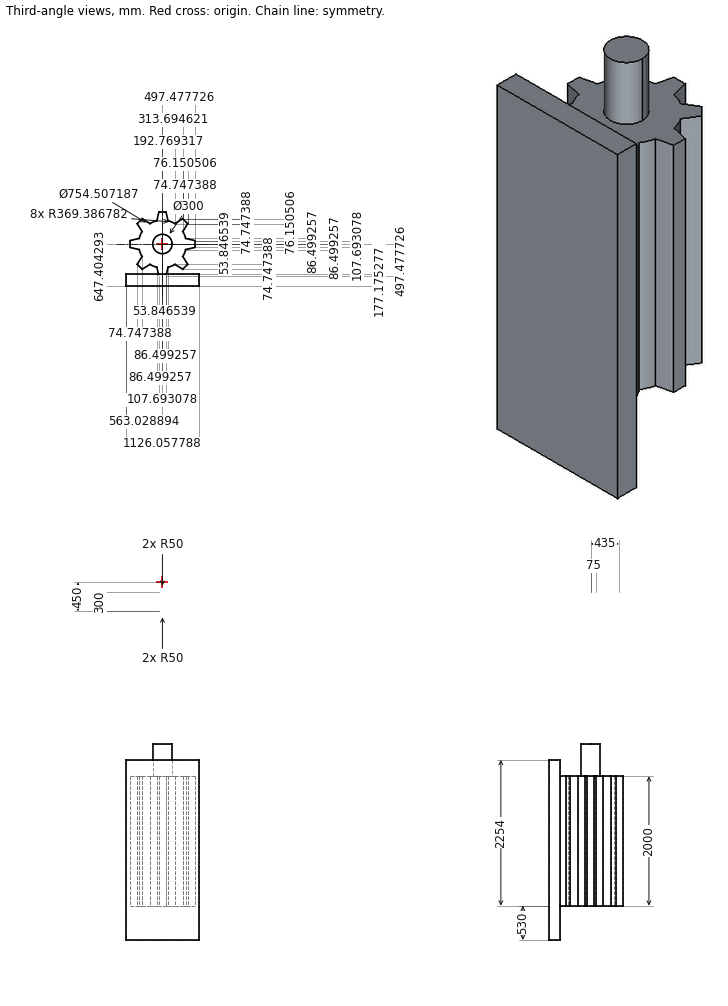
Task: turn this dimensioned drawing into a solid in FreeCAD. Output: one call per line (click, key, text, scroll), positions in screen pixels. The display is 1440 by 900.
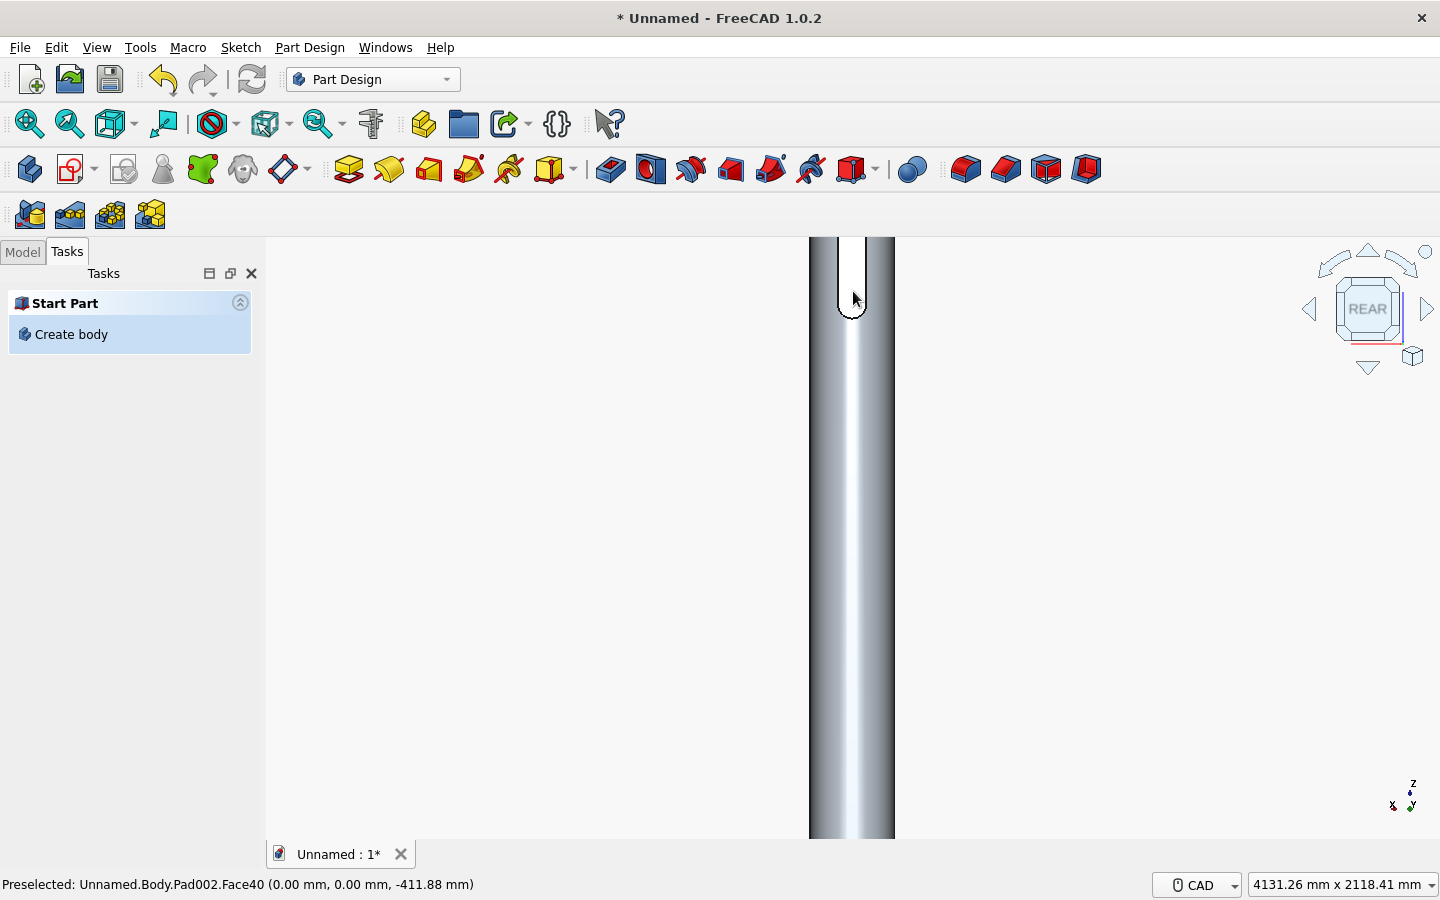
click(852, 293)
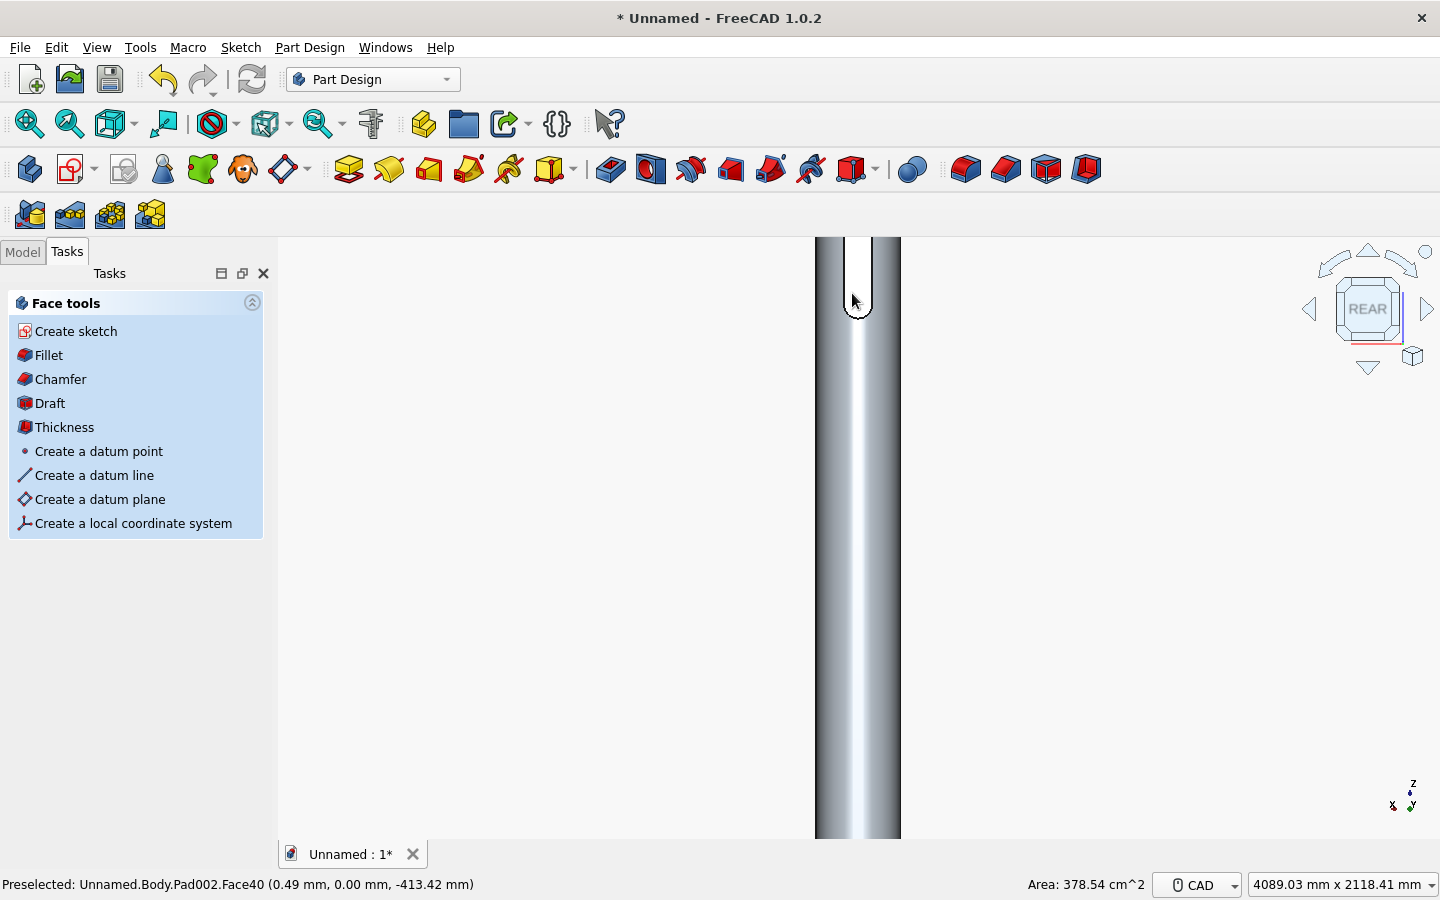
click(70, 170)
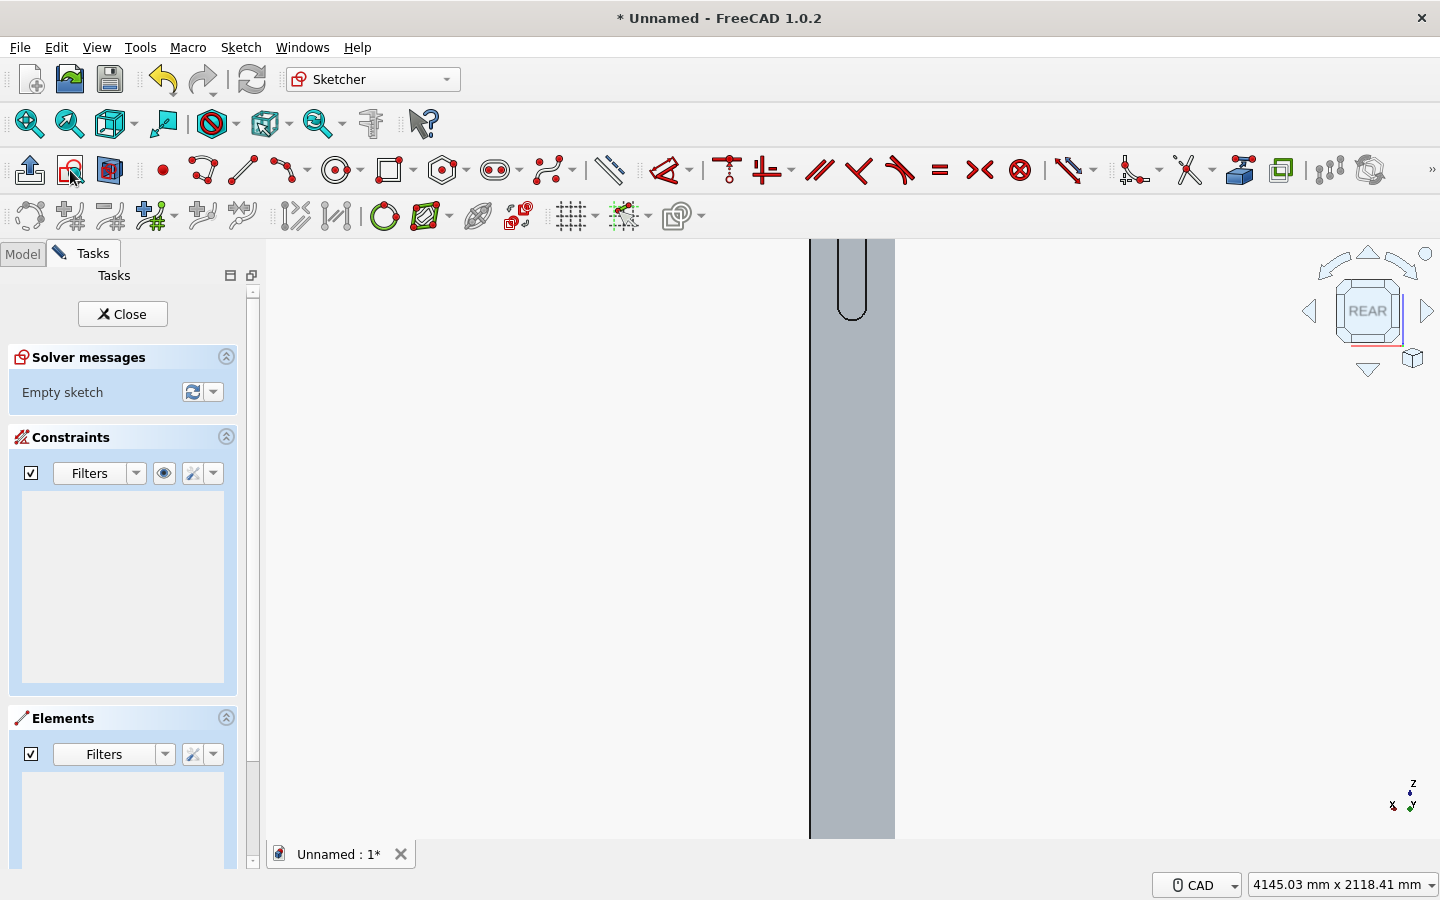
scroll(784, 539, down, 5)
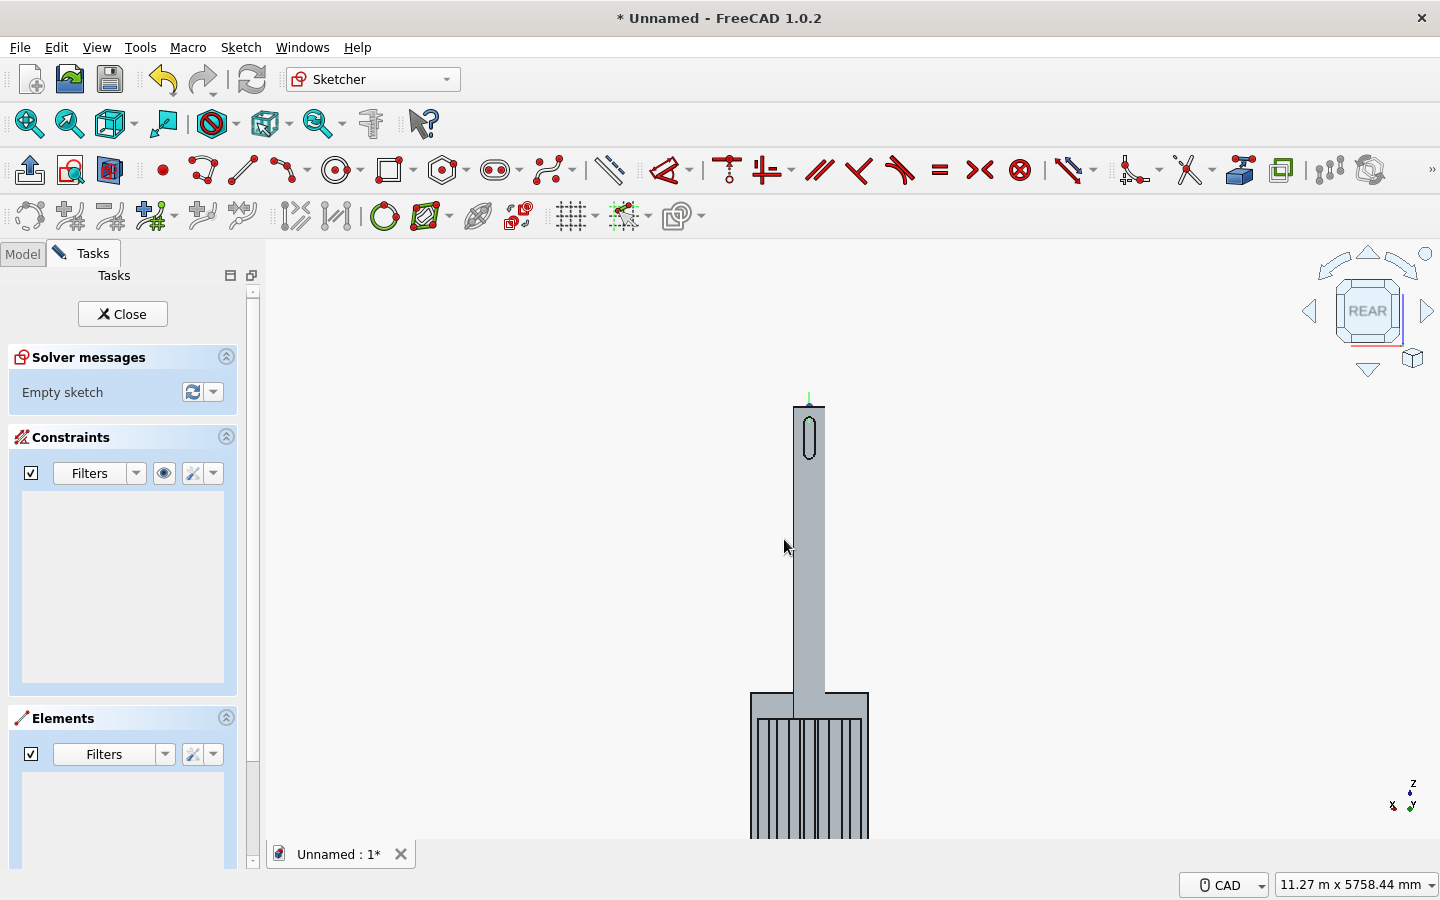
scroll(813, 416, up, 10)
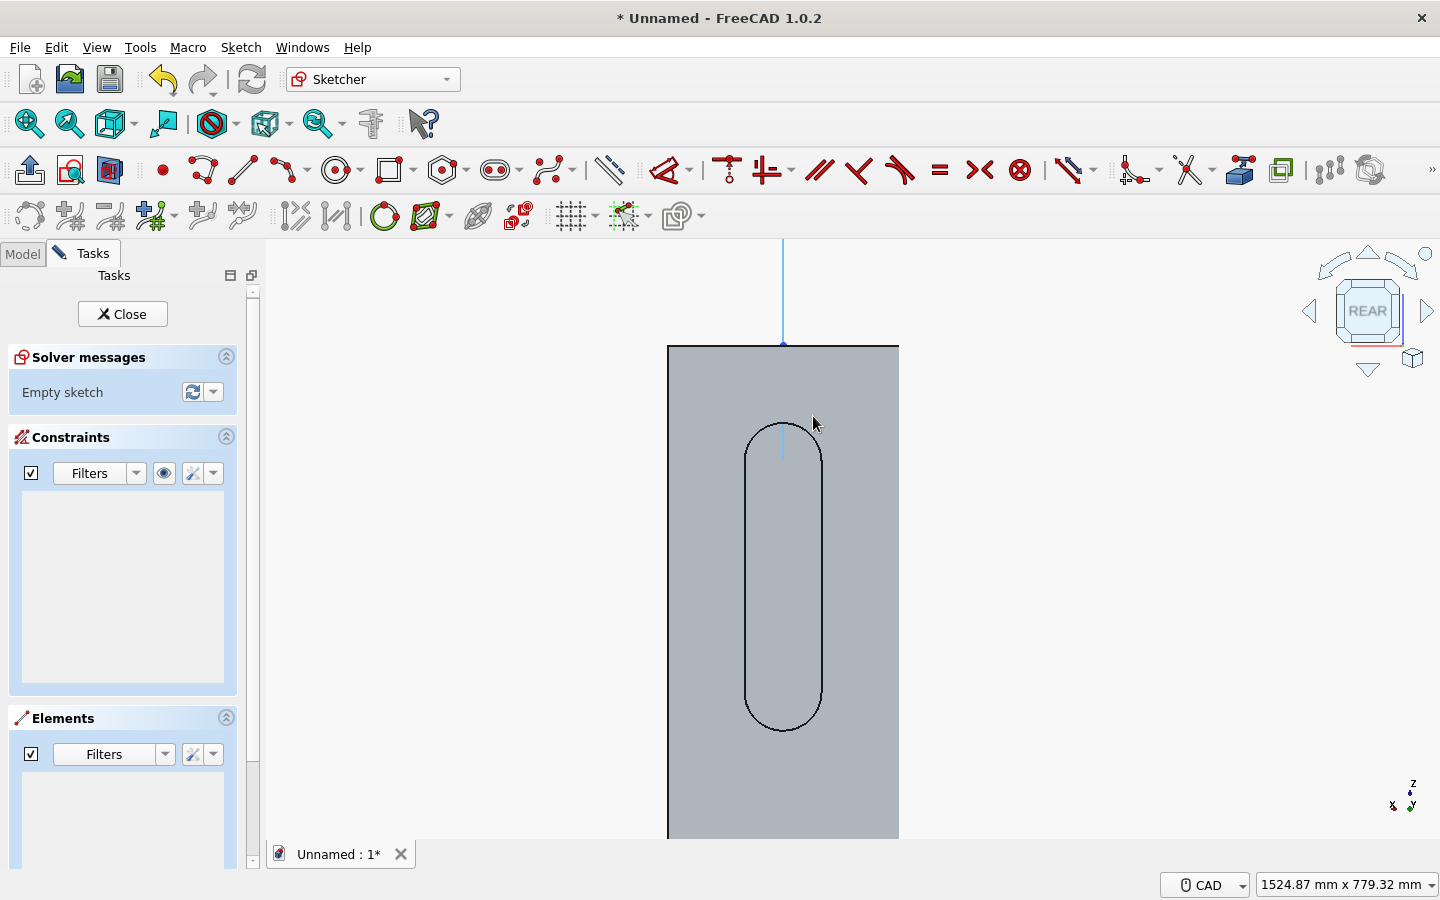
click(496, 170)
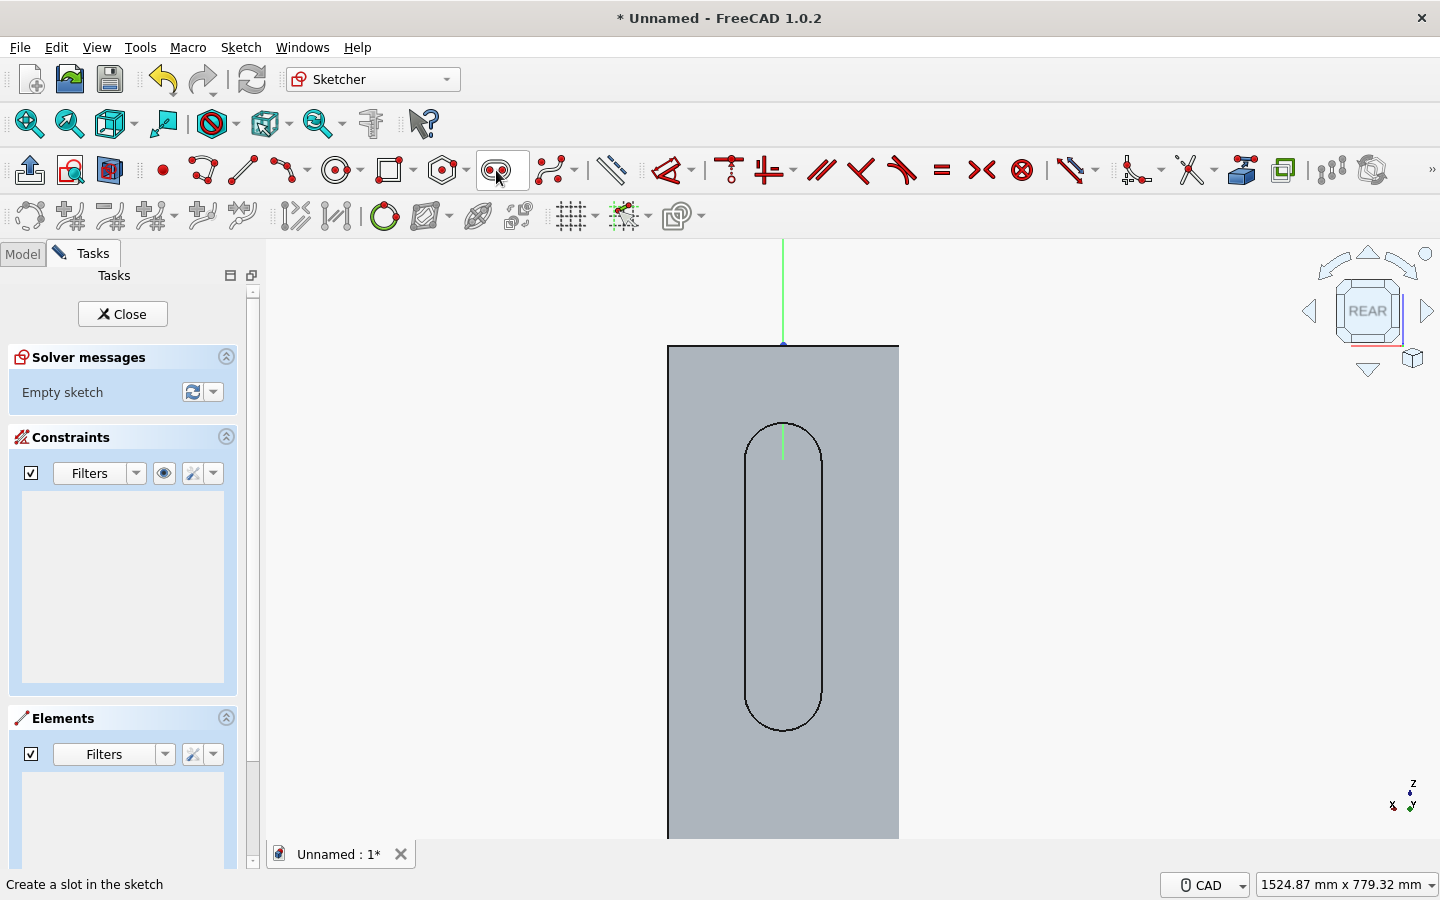
click(783, 692)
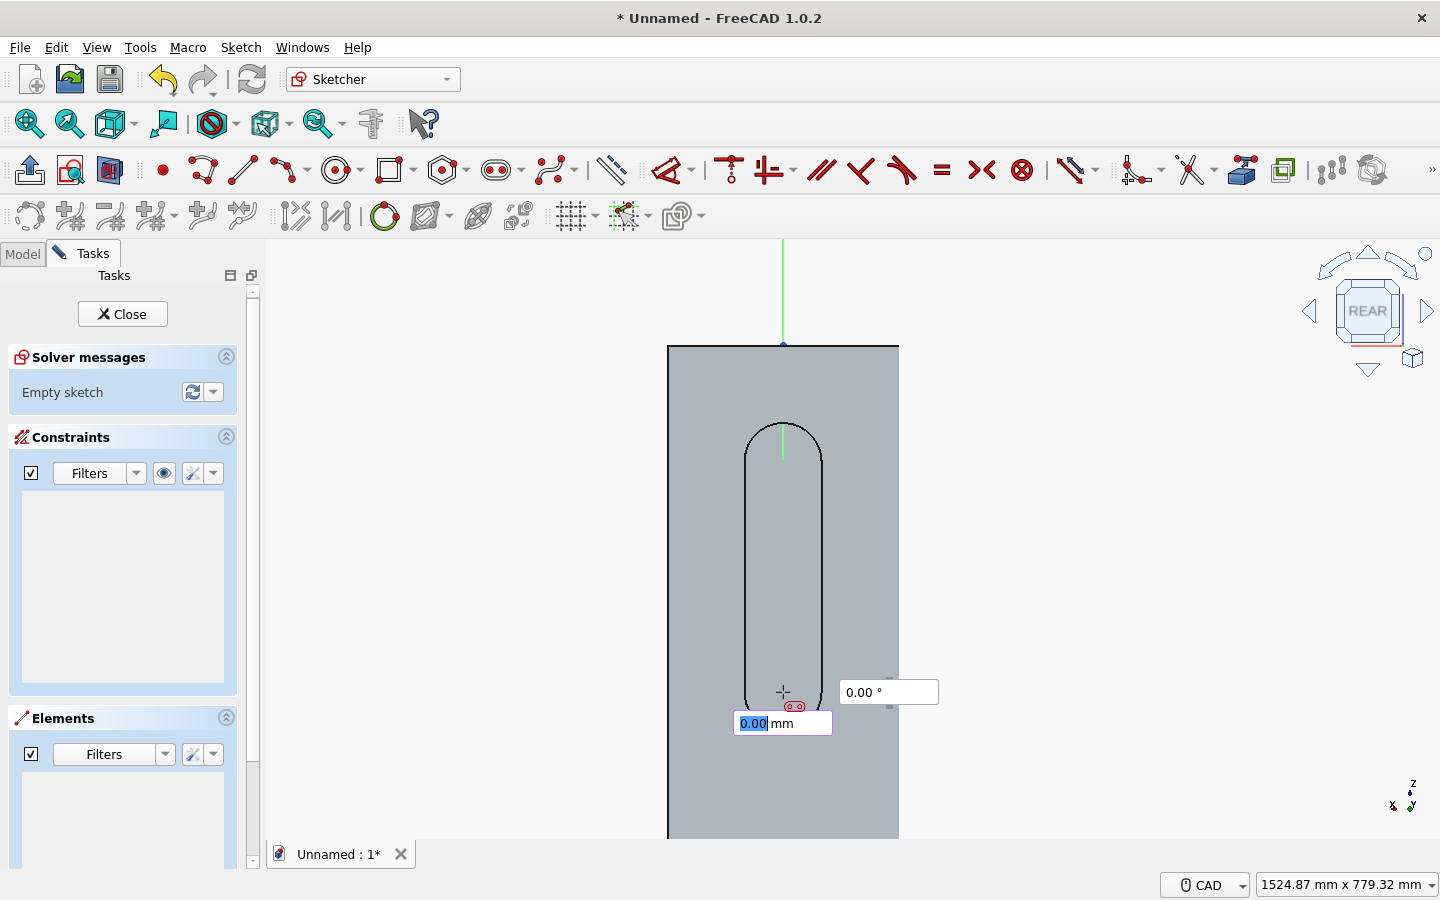
click(792, 461)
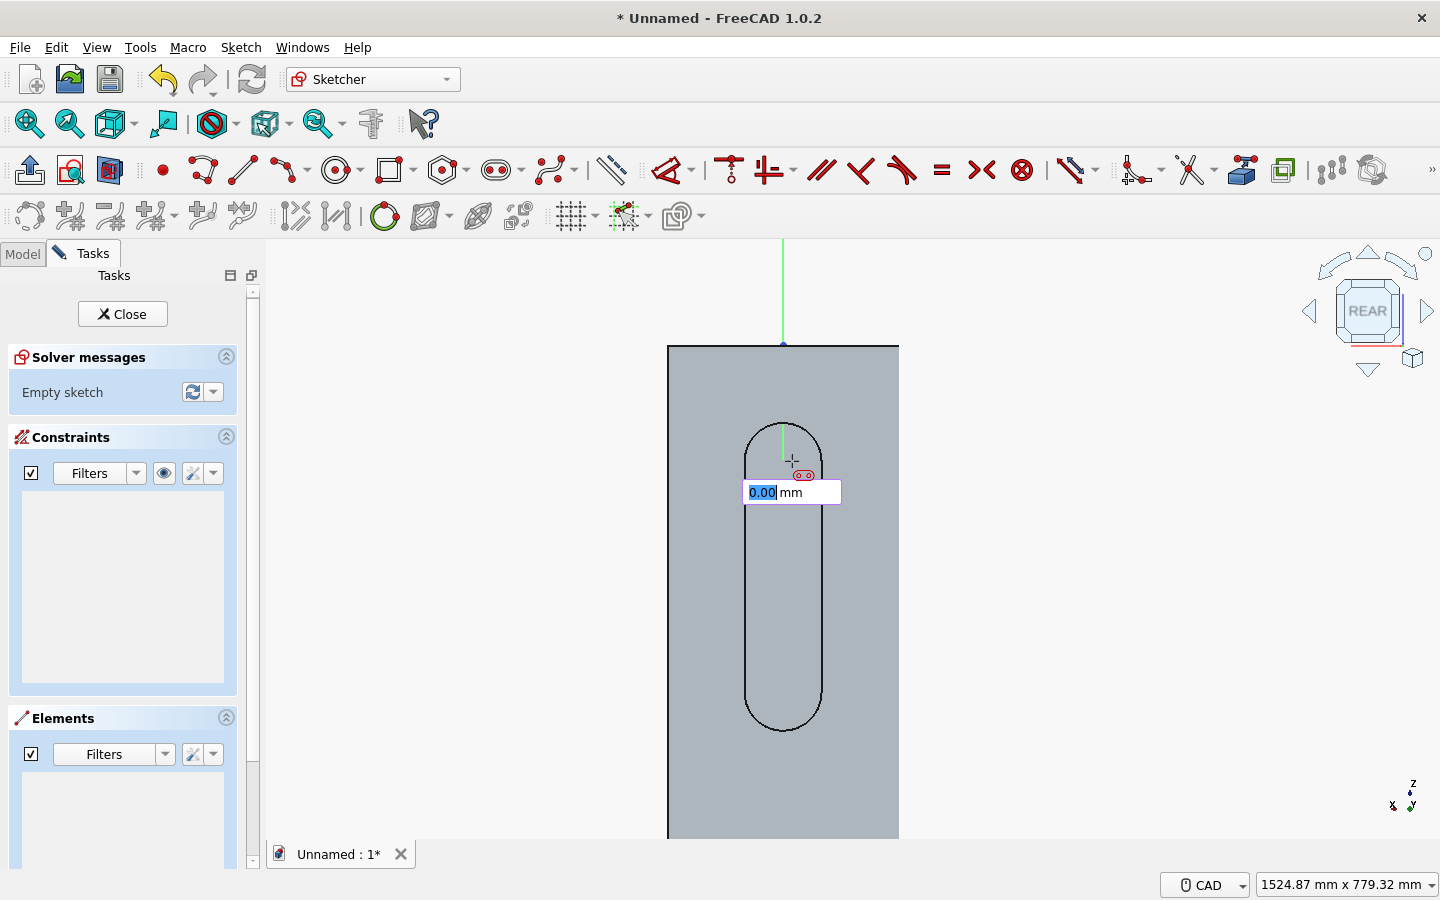
click(745, 577)
key(Escape)